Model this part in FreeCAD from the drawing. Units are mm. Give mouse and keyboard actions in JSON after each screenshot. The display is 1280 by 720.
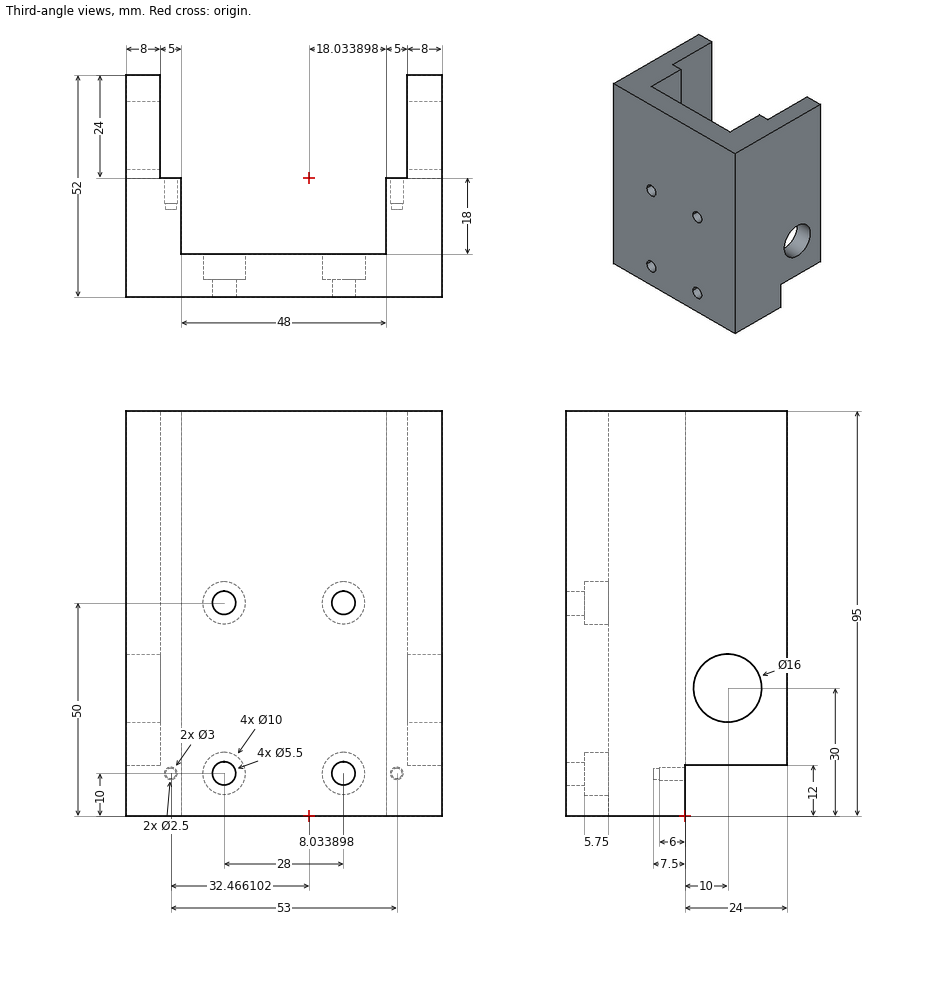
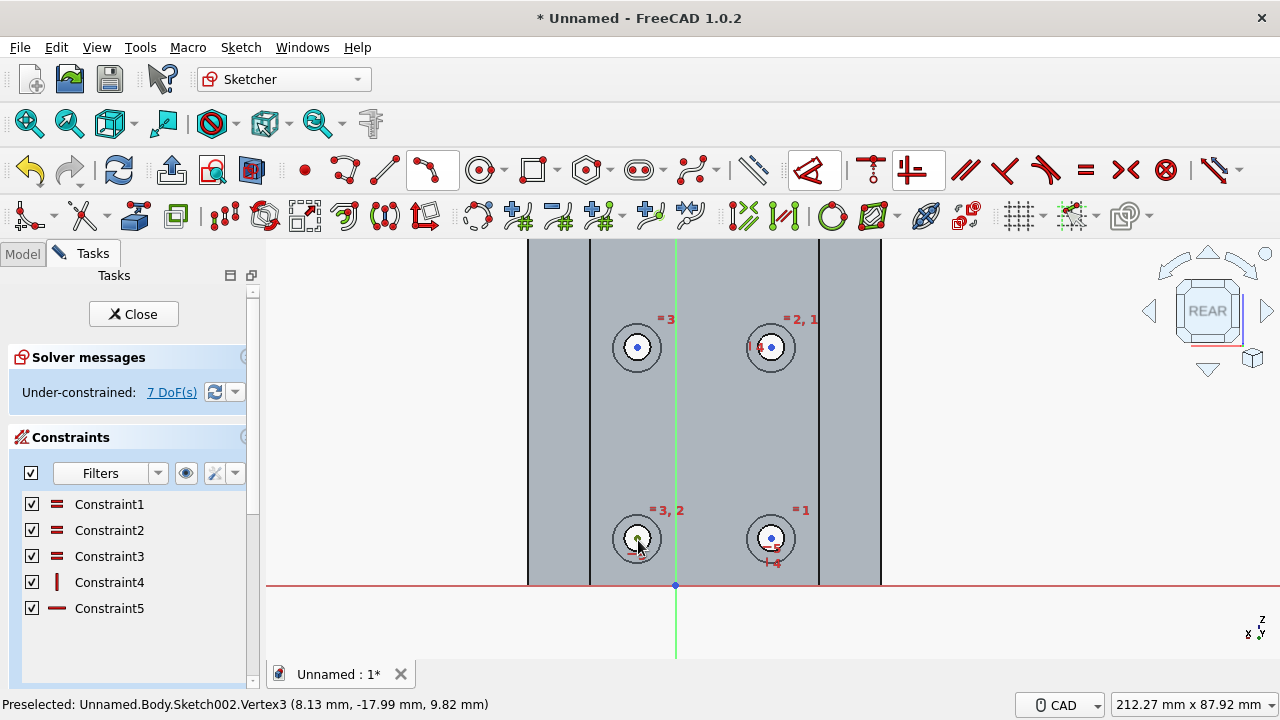
{"action": "left_click", "coordinate": [637, 348]}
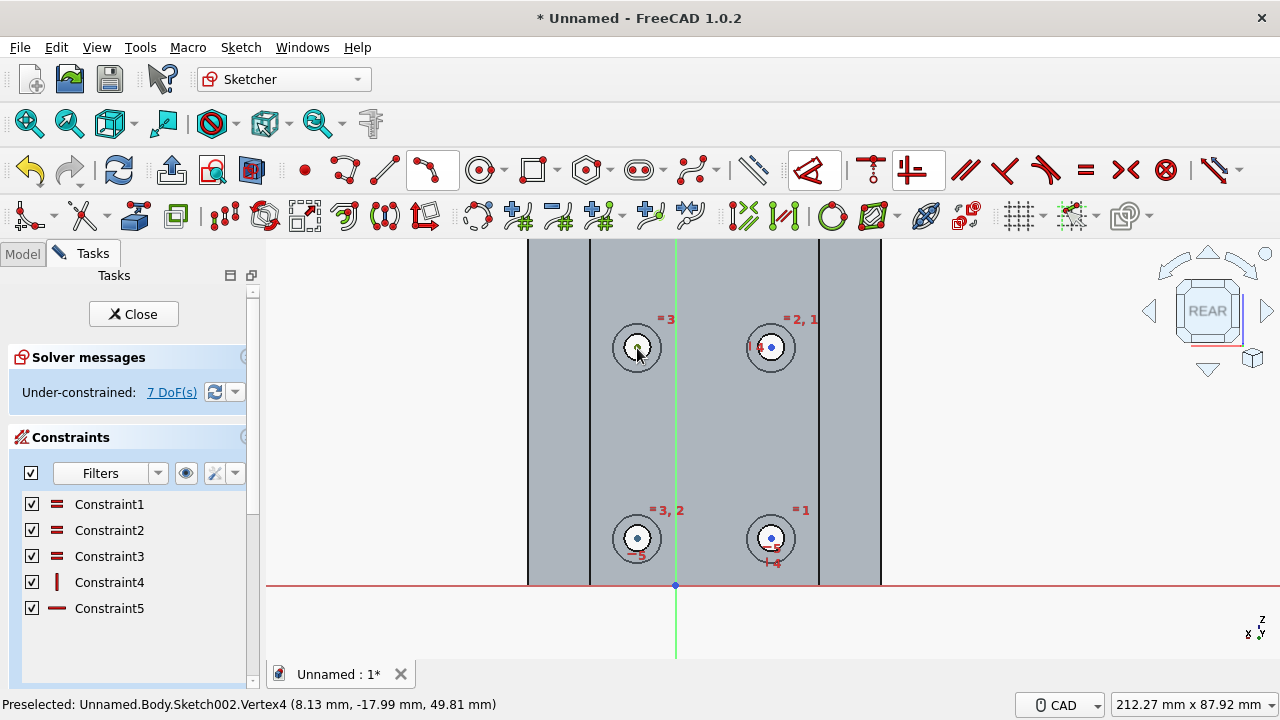
{"action": "key", "text": "v"}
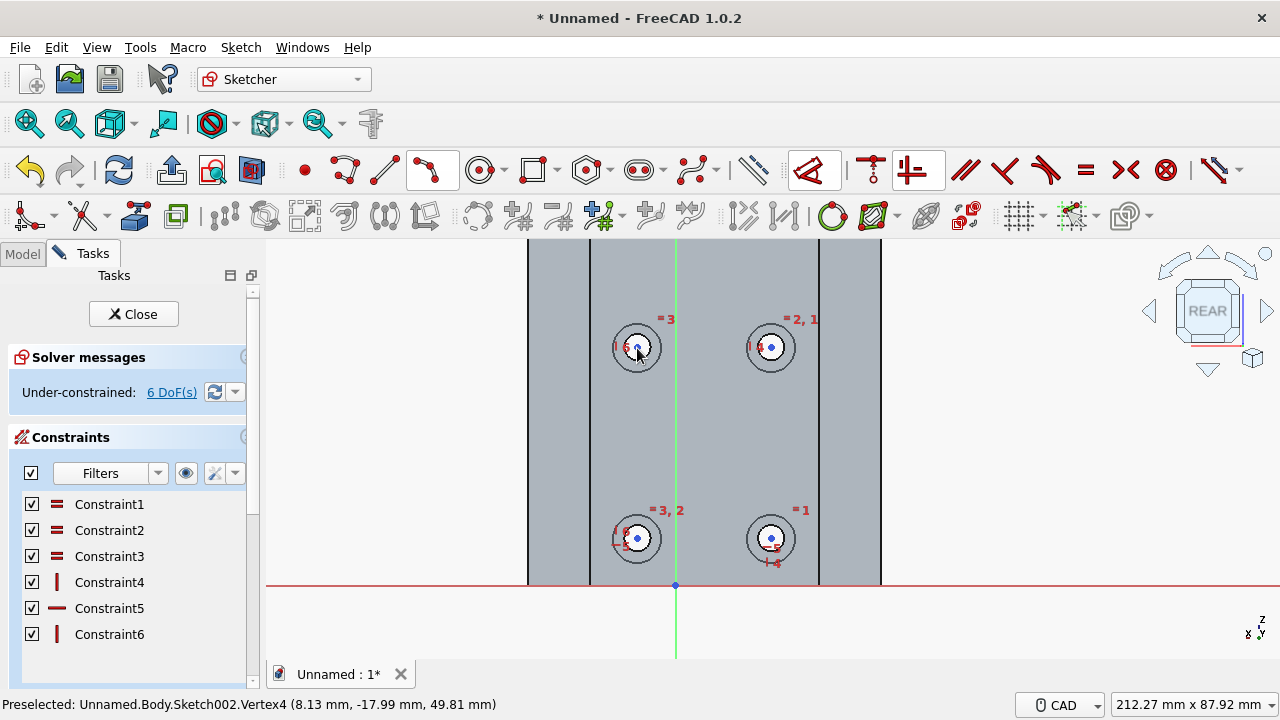
{"action": "left_click", "coordinate": [771, 348]}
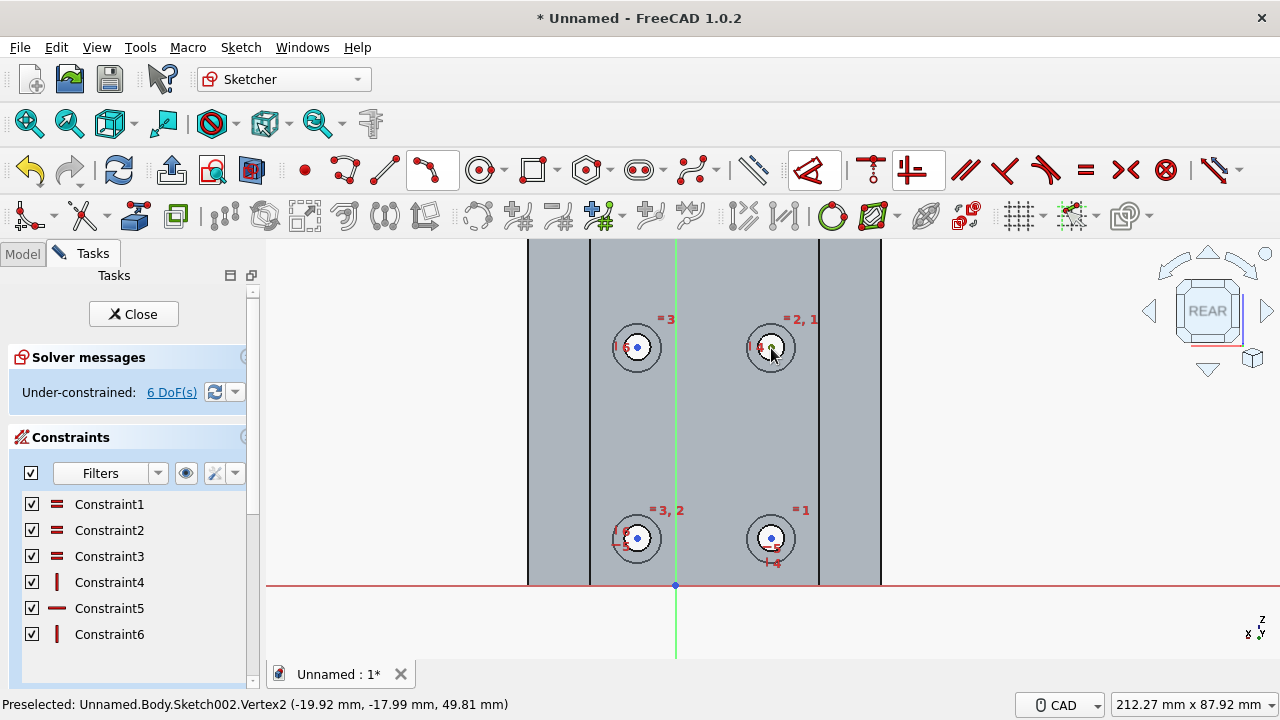
{"action": "left_click", "coordinate": [637, 348]}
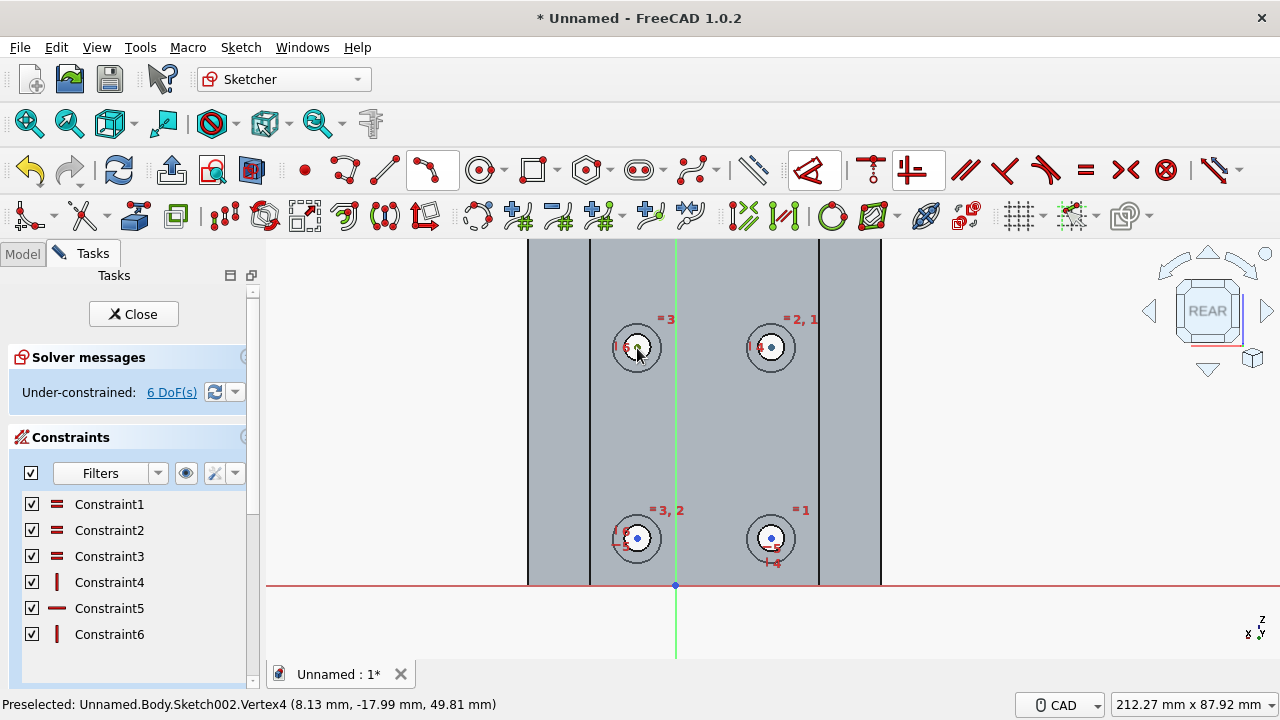
{"action": "left_click", "coordinate": [940, 170]}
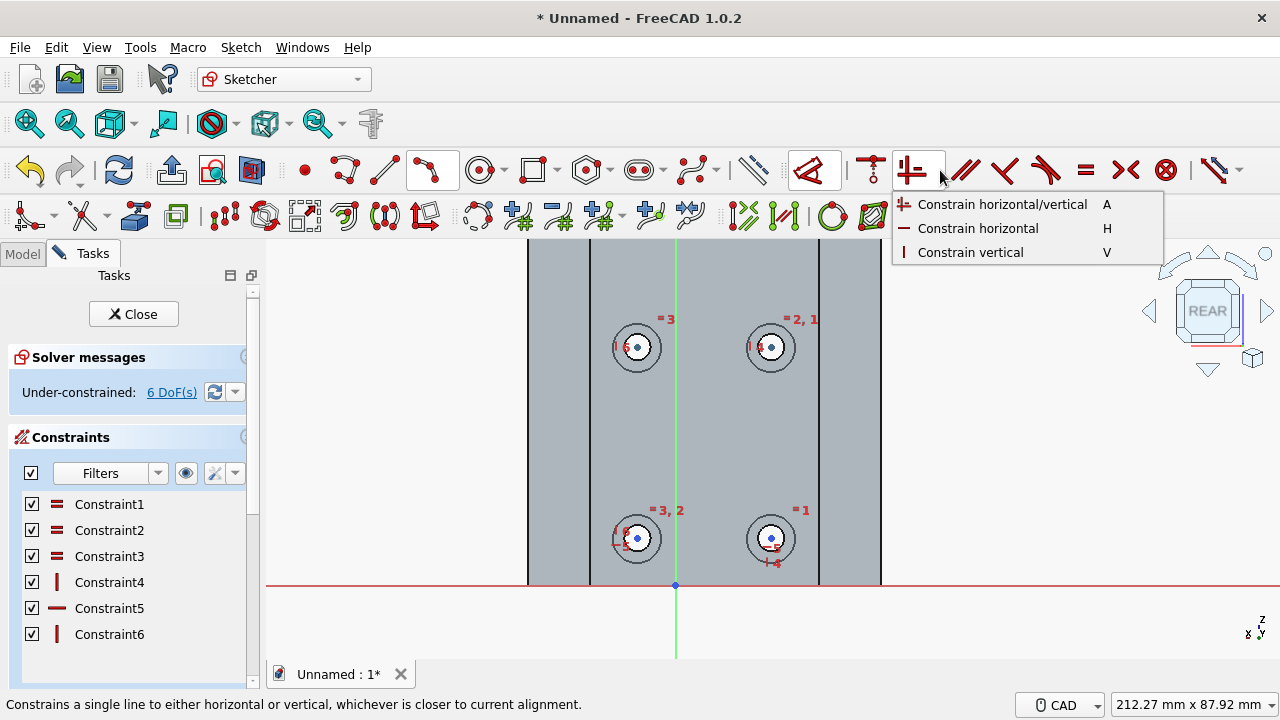
{"action": "left_click", "coordinate": [1028, 228]}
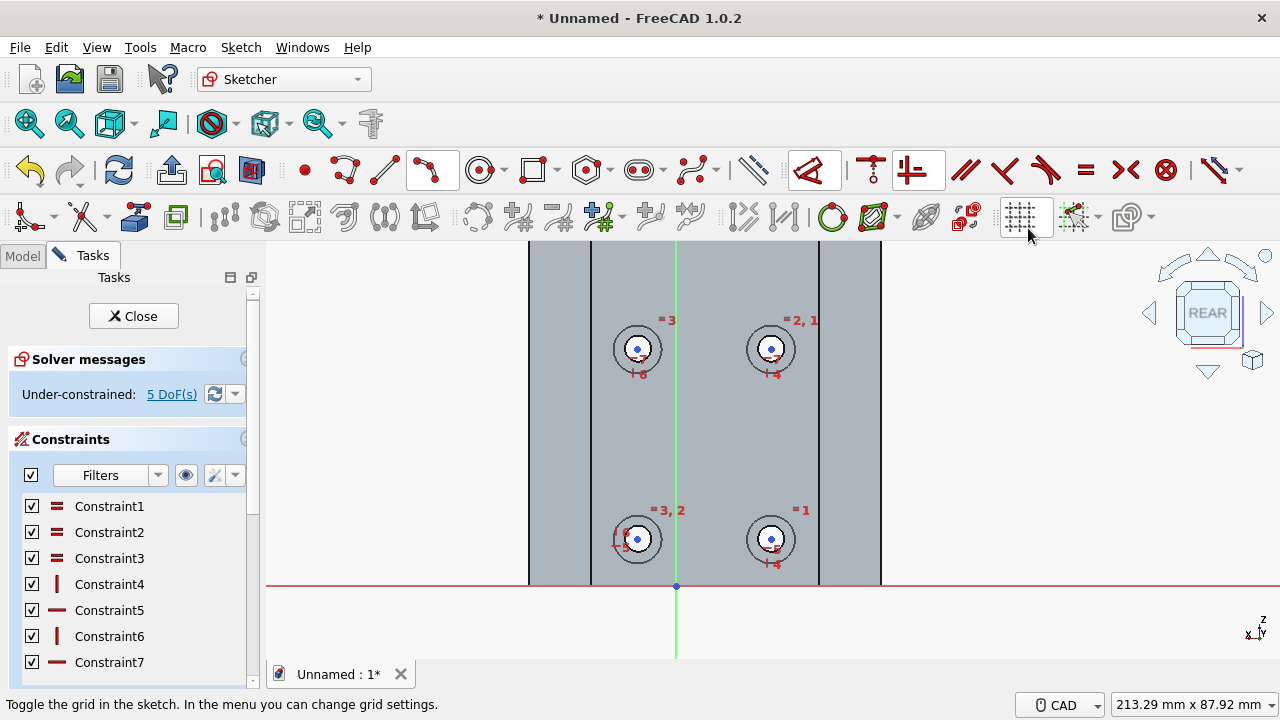
{"action": "left_click", "coordinate": [788, 523]}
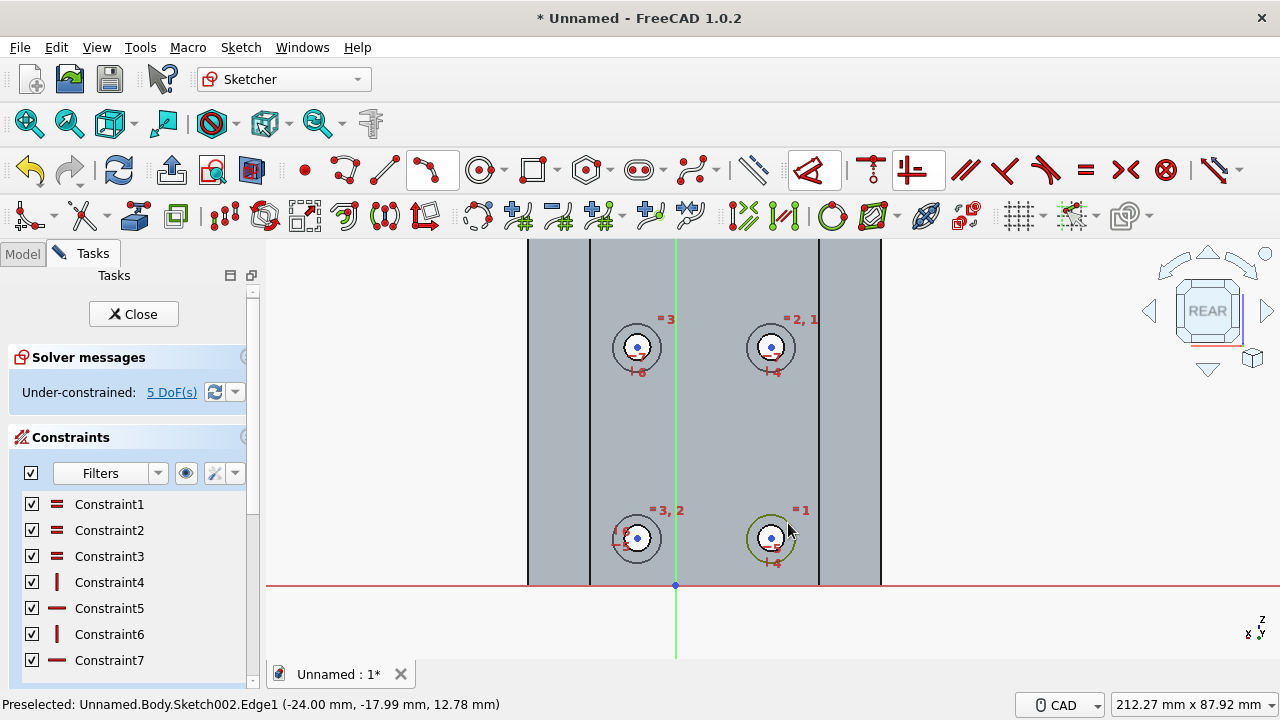
{"action": "key", "text": "k o"}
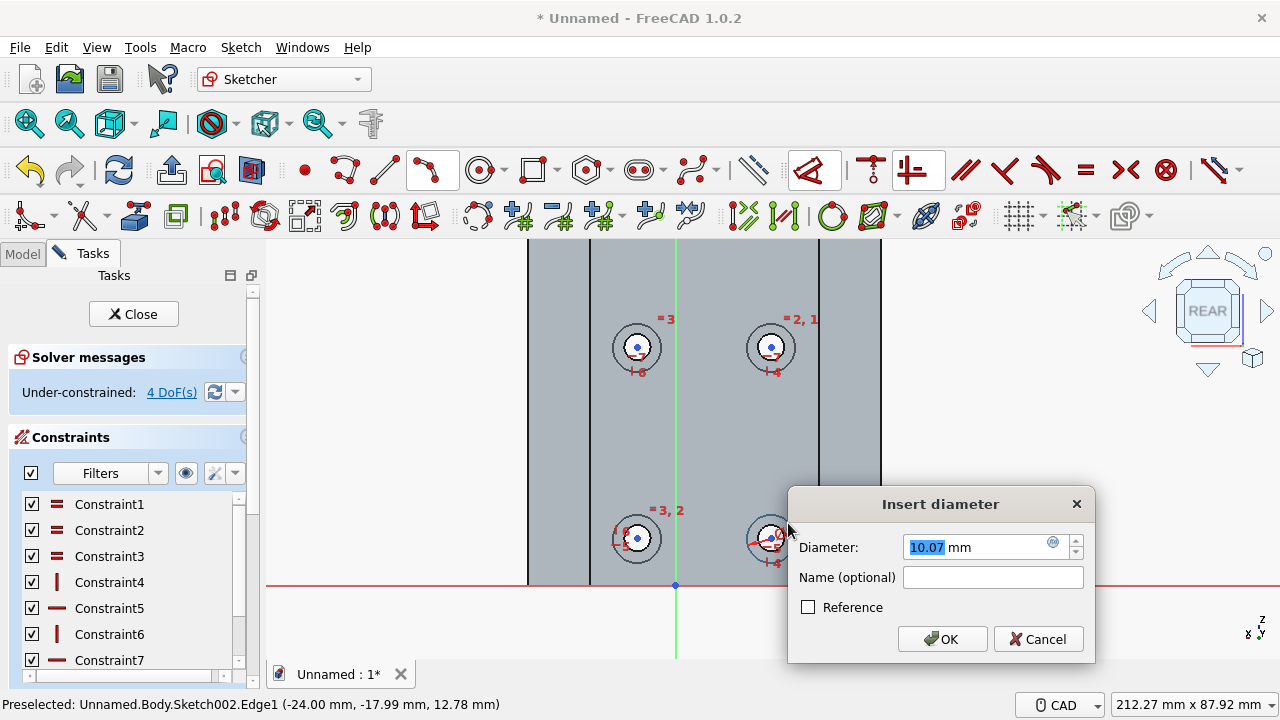
{"action": "type", "text": "10"}
{"action": "key", "text": "Return"}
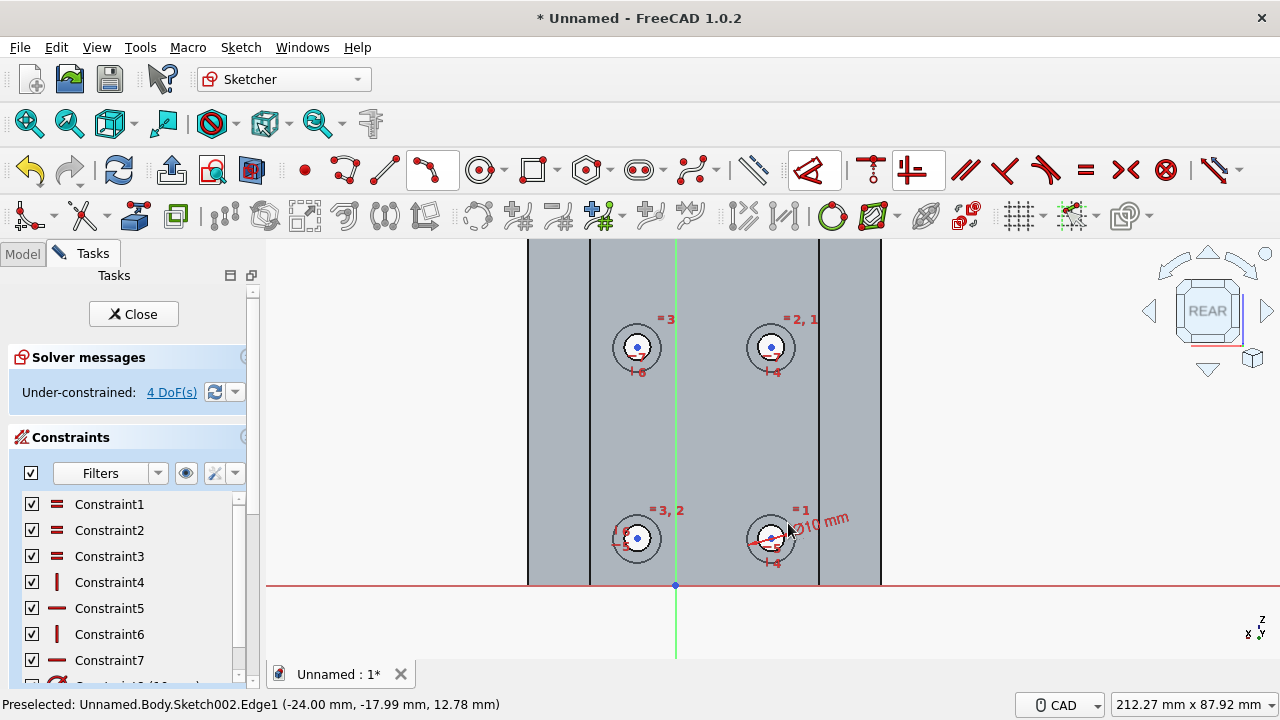
{"action": "left_click", "coordinate": [771, 539]}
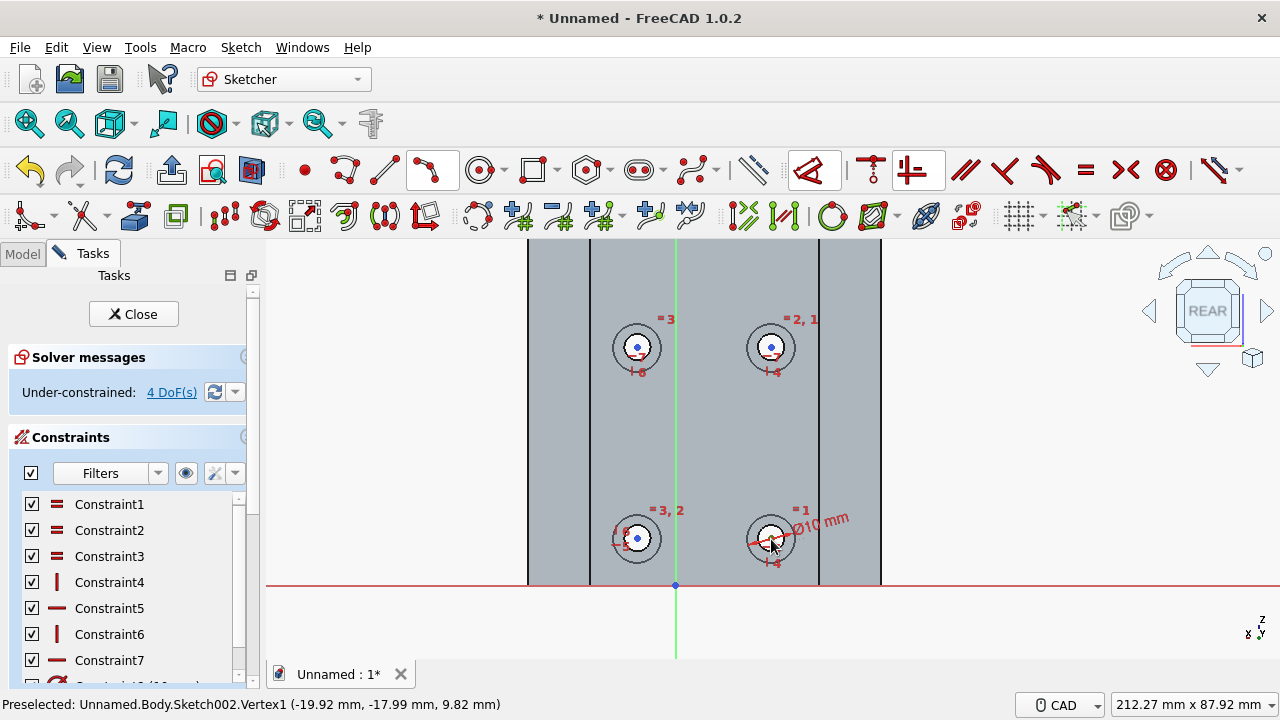
{"action": "key", "text": "i"}